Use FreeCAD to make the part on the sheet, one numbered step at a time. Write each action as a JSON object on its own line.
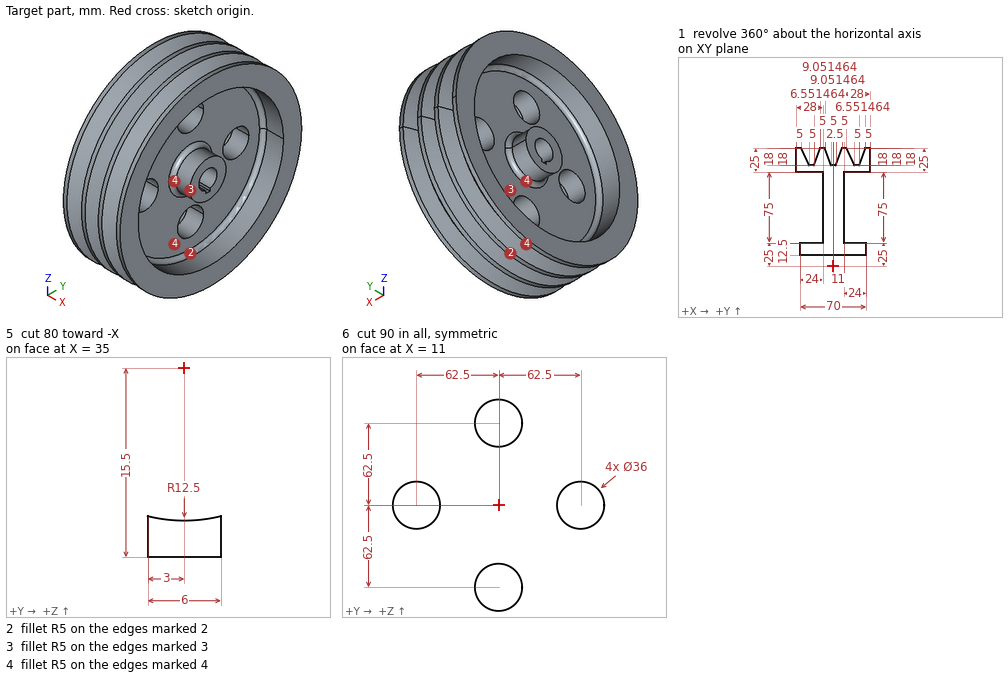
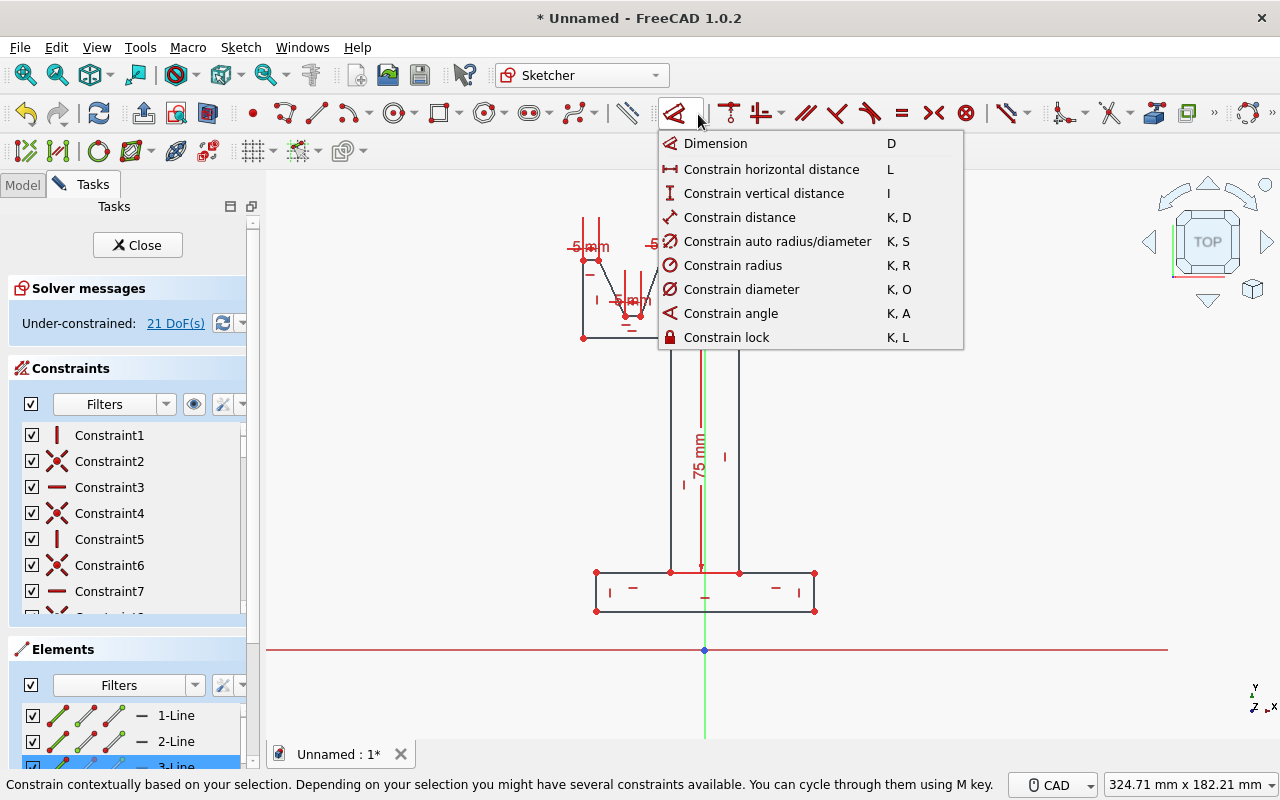
{"action": "left_click", "coordinate": [811, 193]}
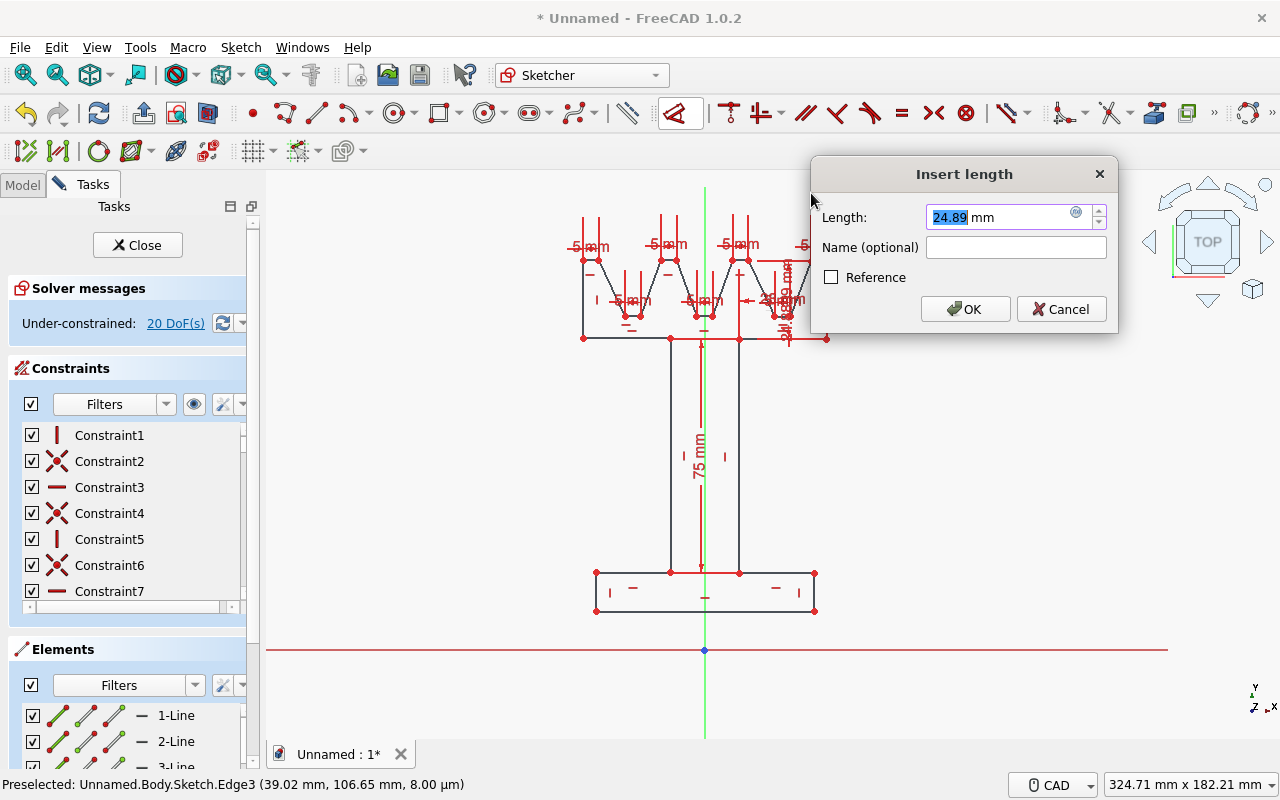
{"action": "type", "text": "25"}
{"action": "key", "text": "Return"}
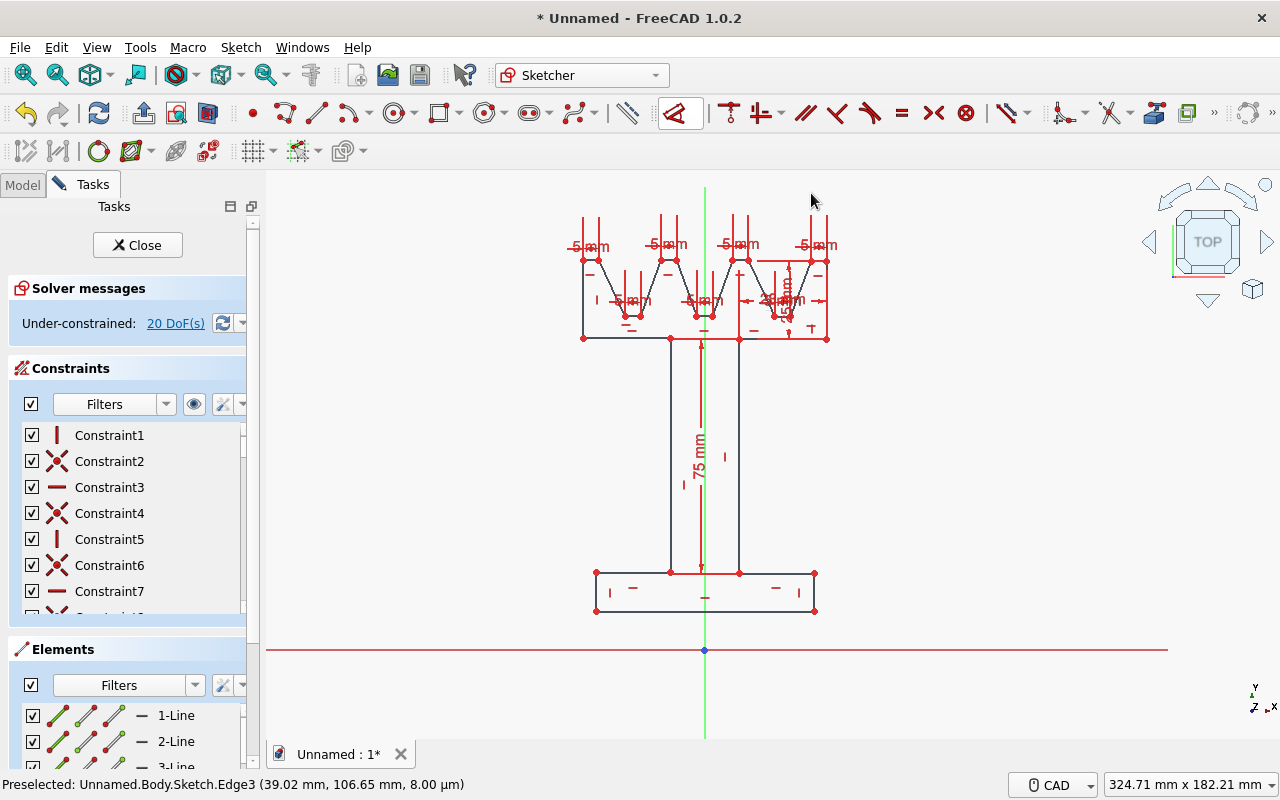
{"action": "left_click", "coordinate": [583, 284]}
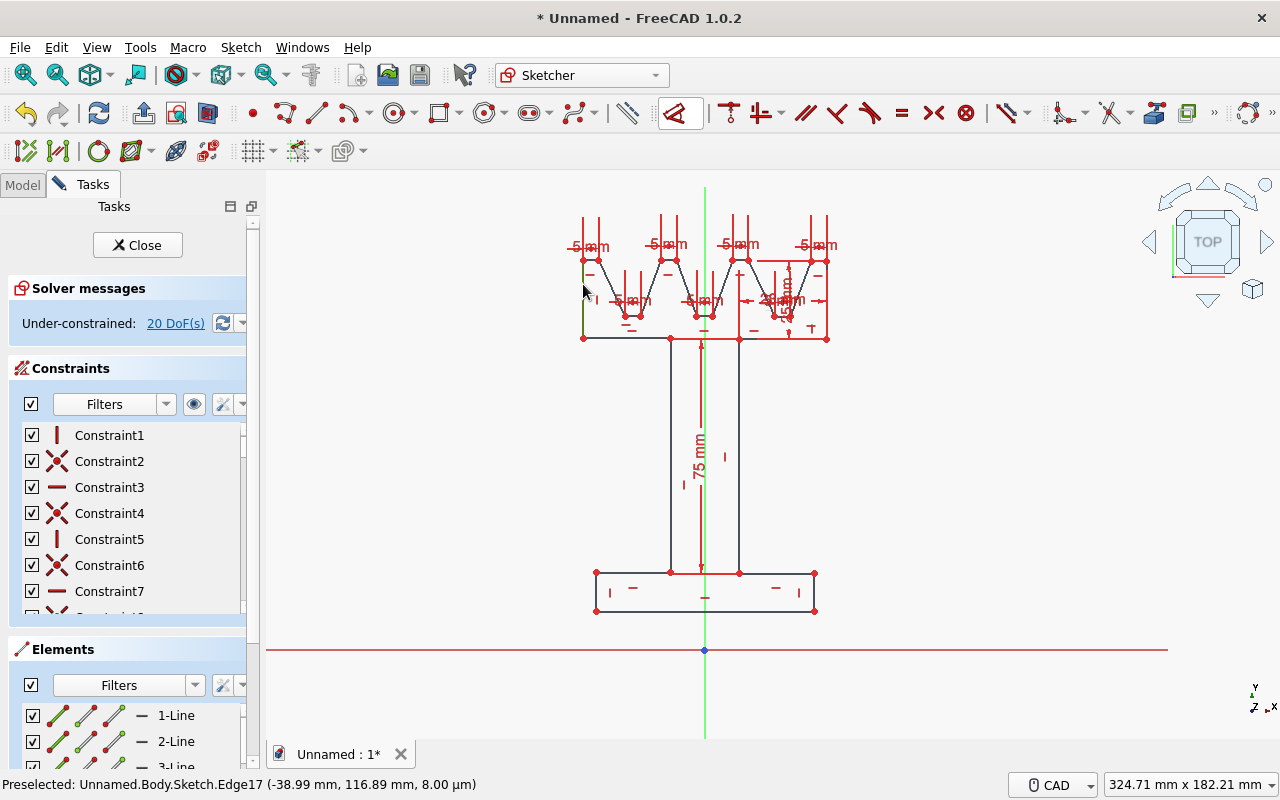
{"action": "left_click", "coordinate": [698, 114]}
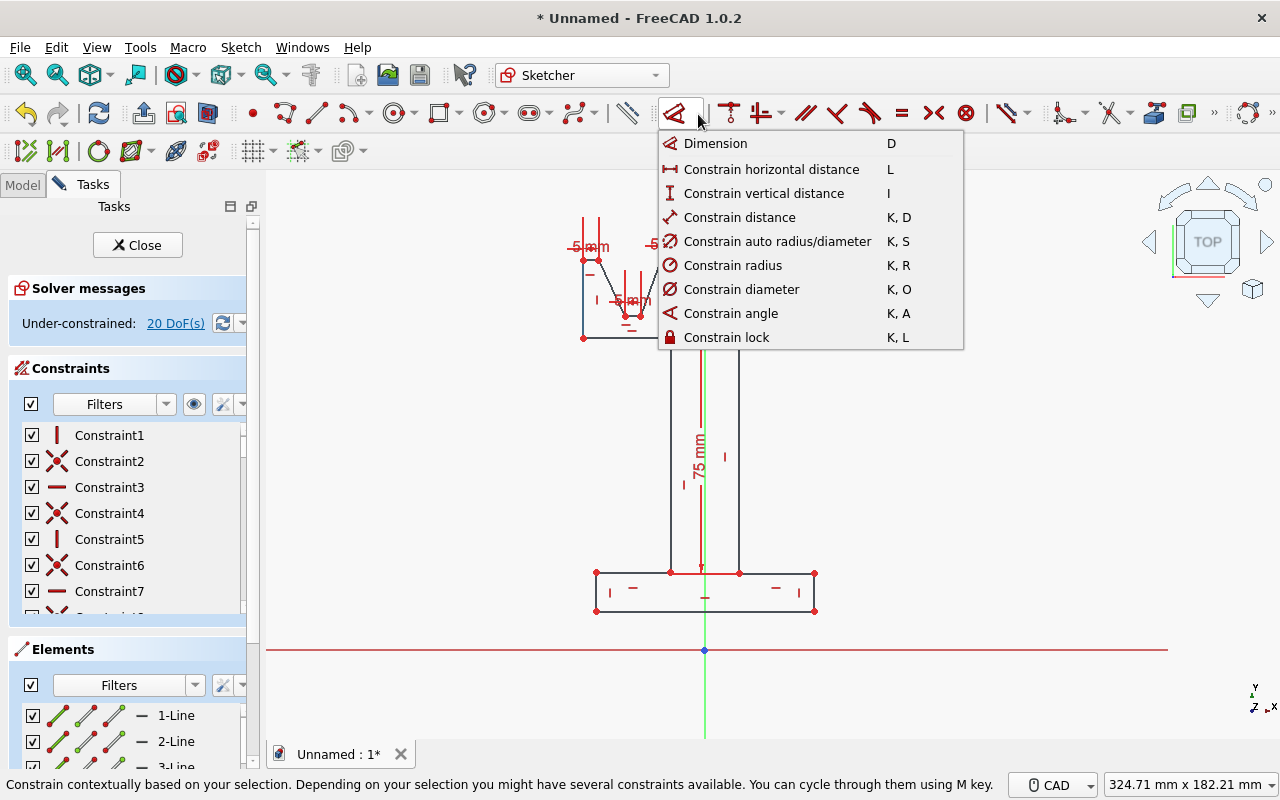
{"action": "left_click", "coordinate": [811, 193]}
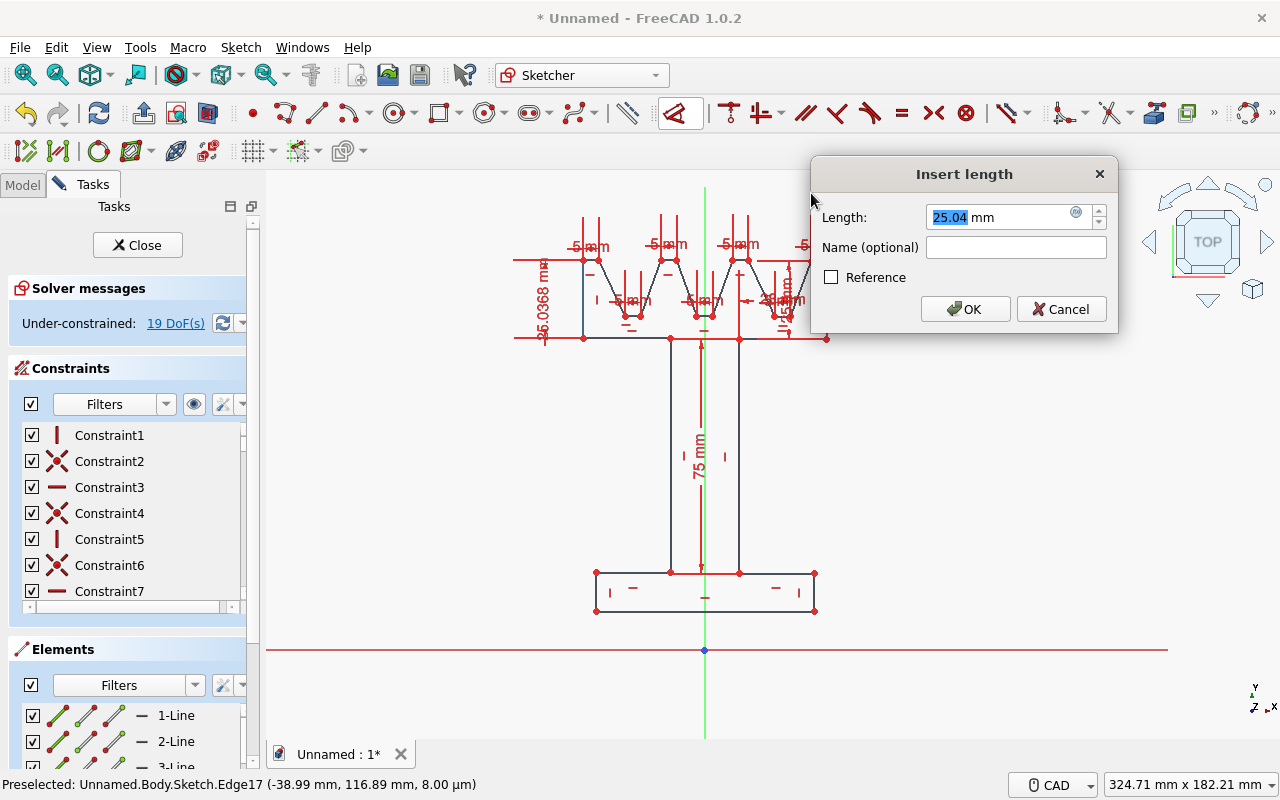
{"action": "type", "text": "25"}
{"action": "key", "text": "Return"}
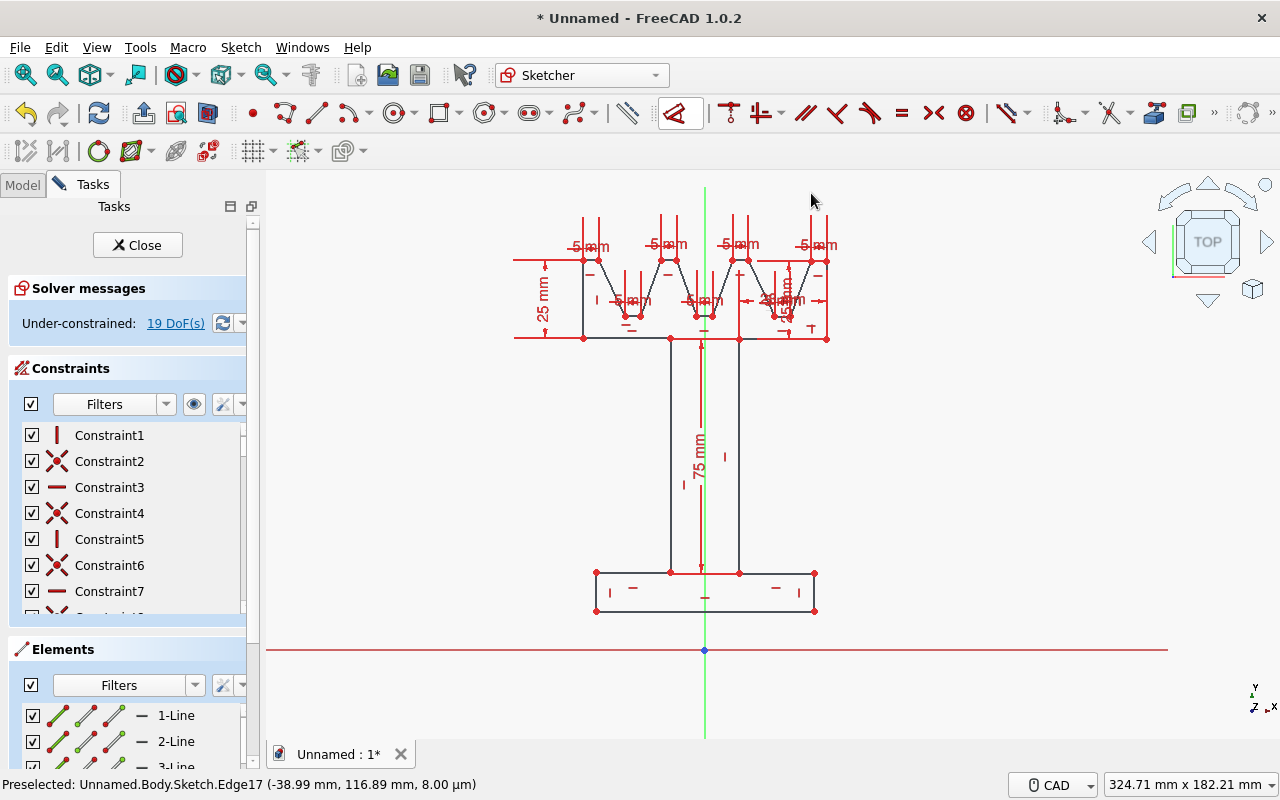
{"action": "left_click", "coordinate": [609, 338]}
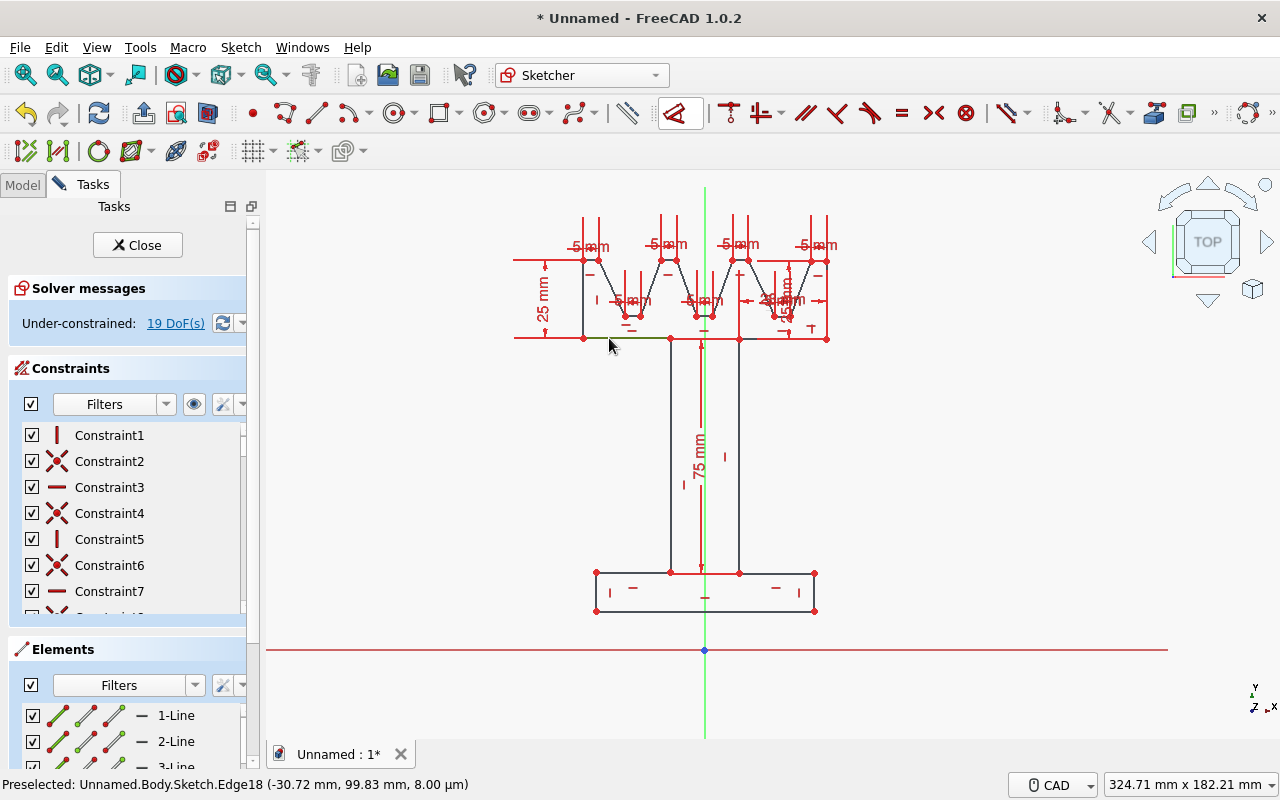
{"action": "left_click", "coordinate": [698, 114]}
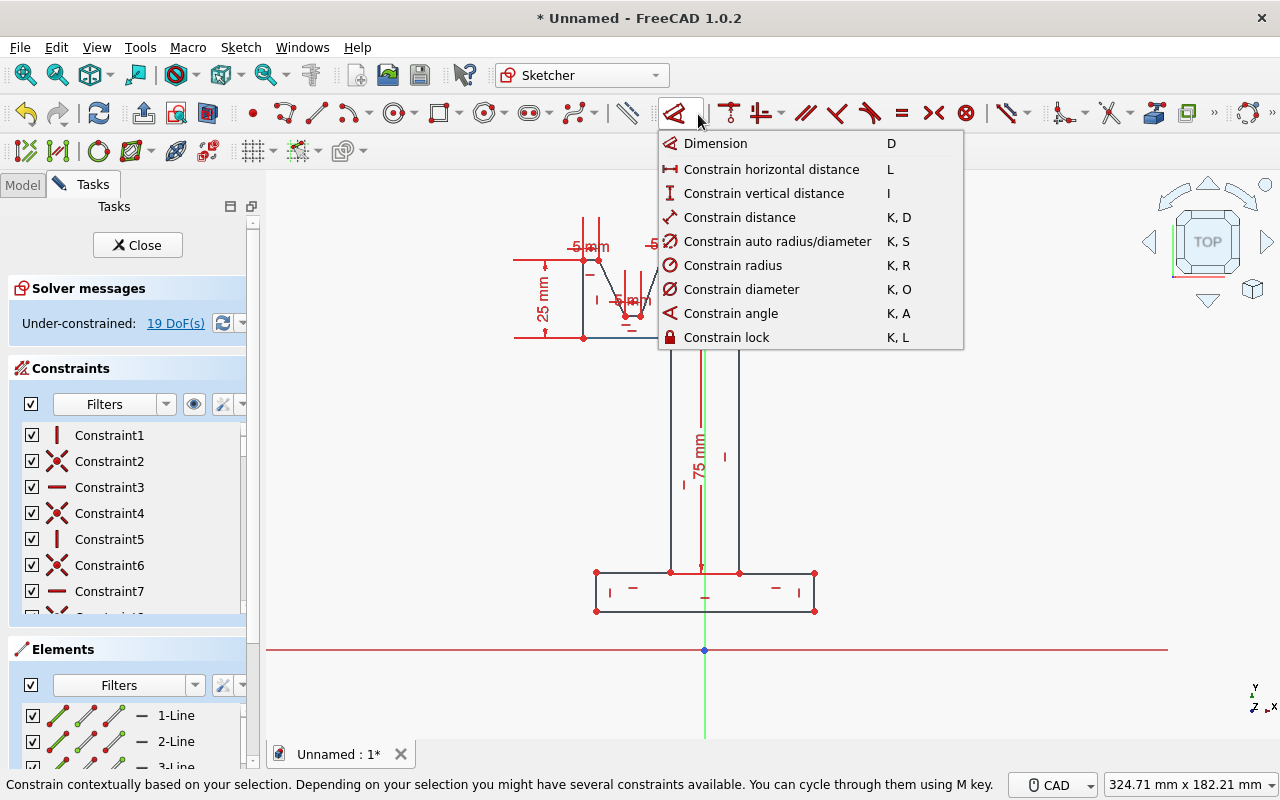
{"action": "left_click", "coordinate": [811, 169]}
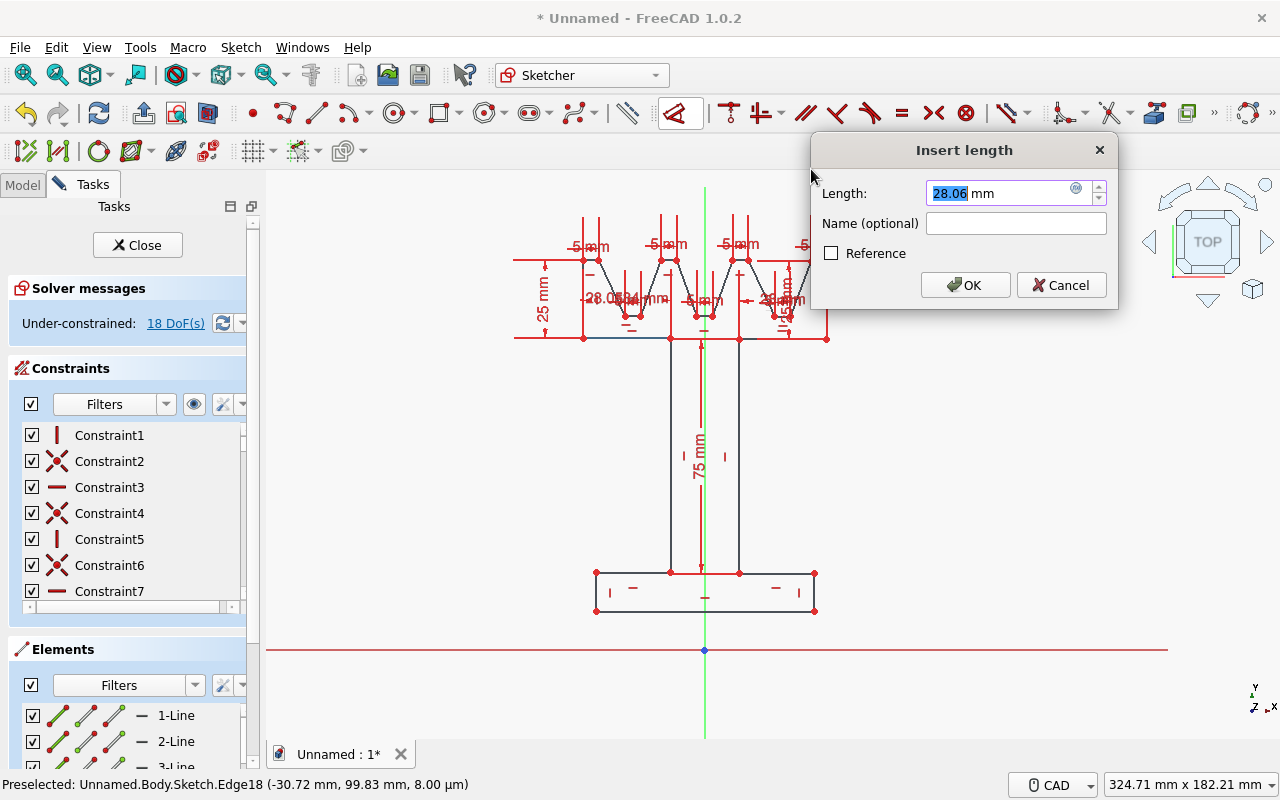
{"action": "type", "text": "28"}
{"action": "key", "text": "Return"}